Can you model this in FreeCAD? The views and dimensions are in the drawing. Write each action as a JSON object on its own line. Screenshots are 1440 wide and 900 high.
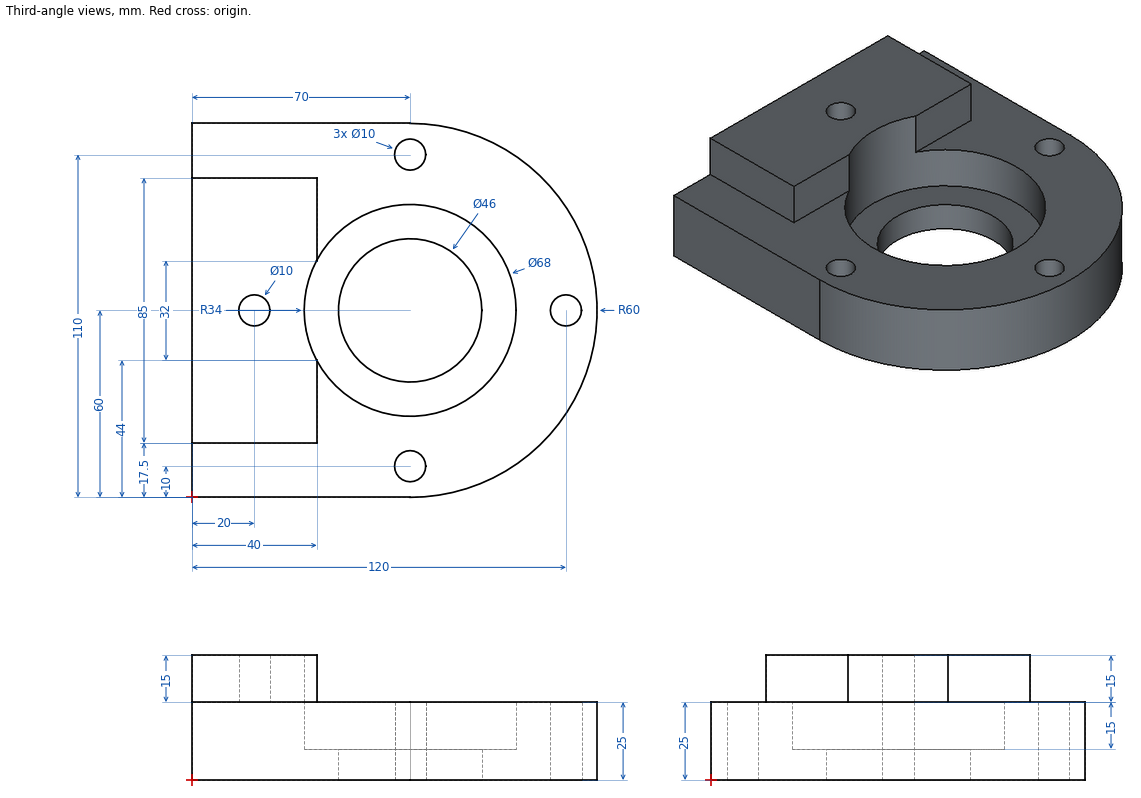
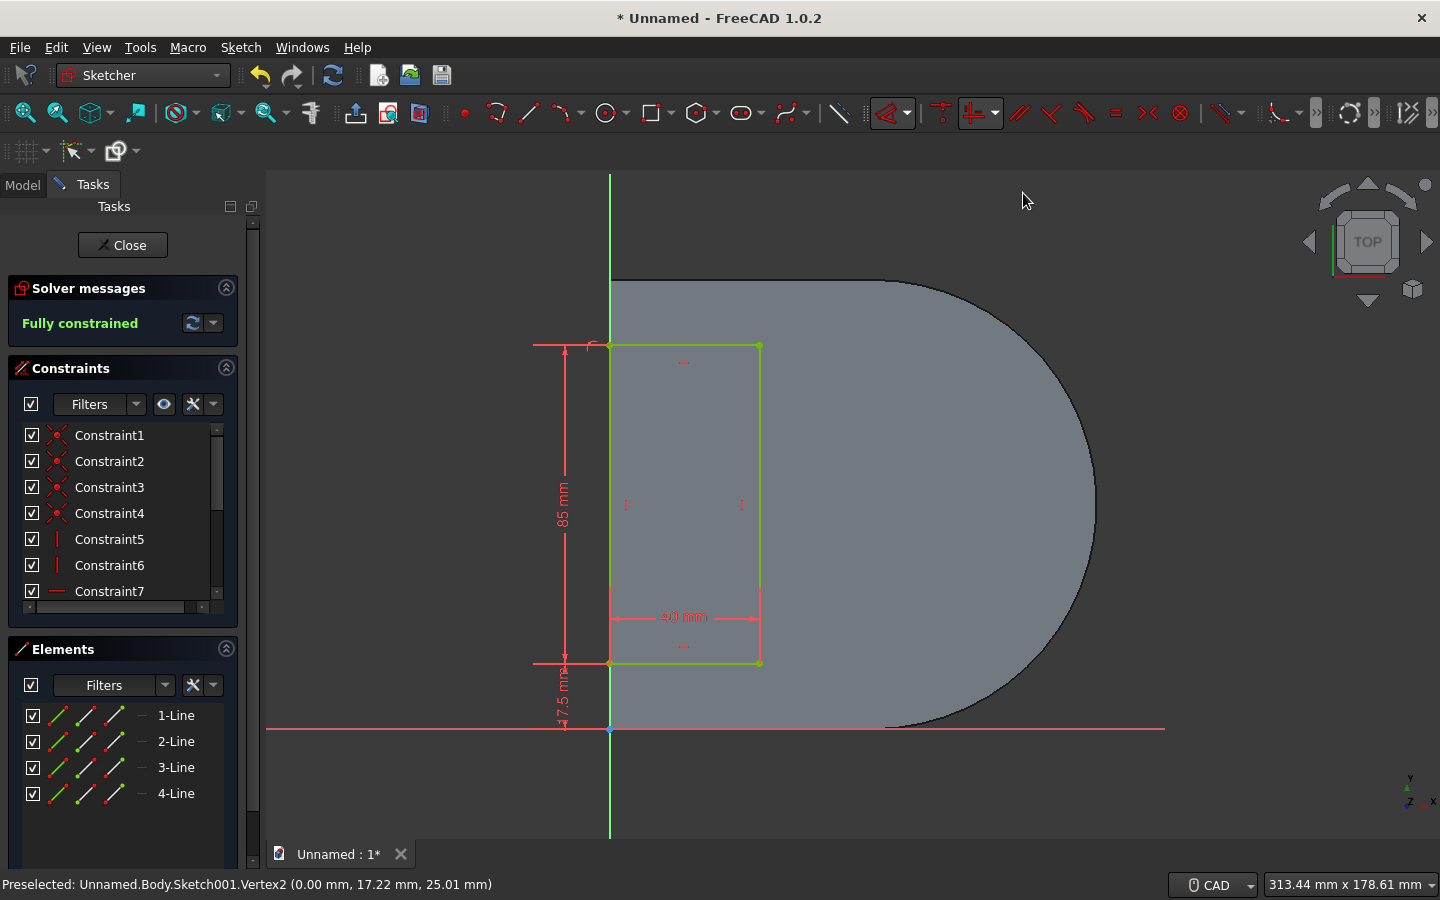
{"action": "left_click", "coordinate": [123, 245]}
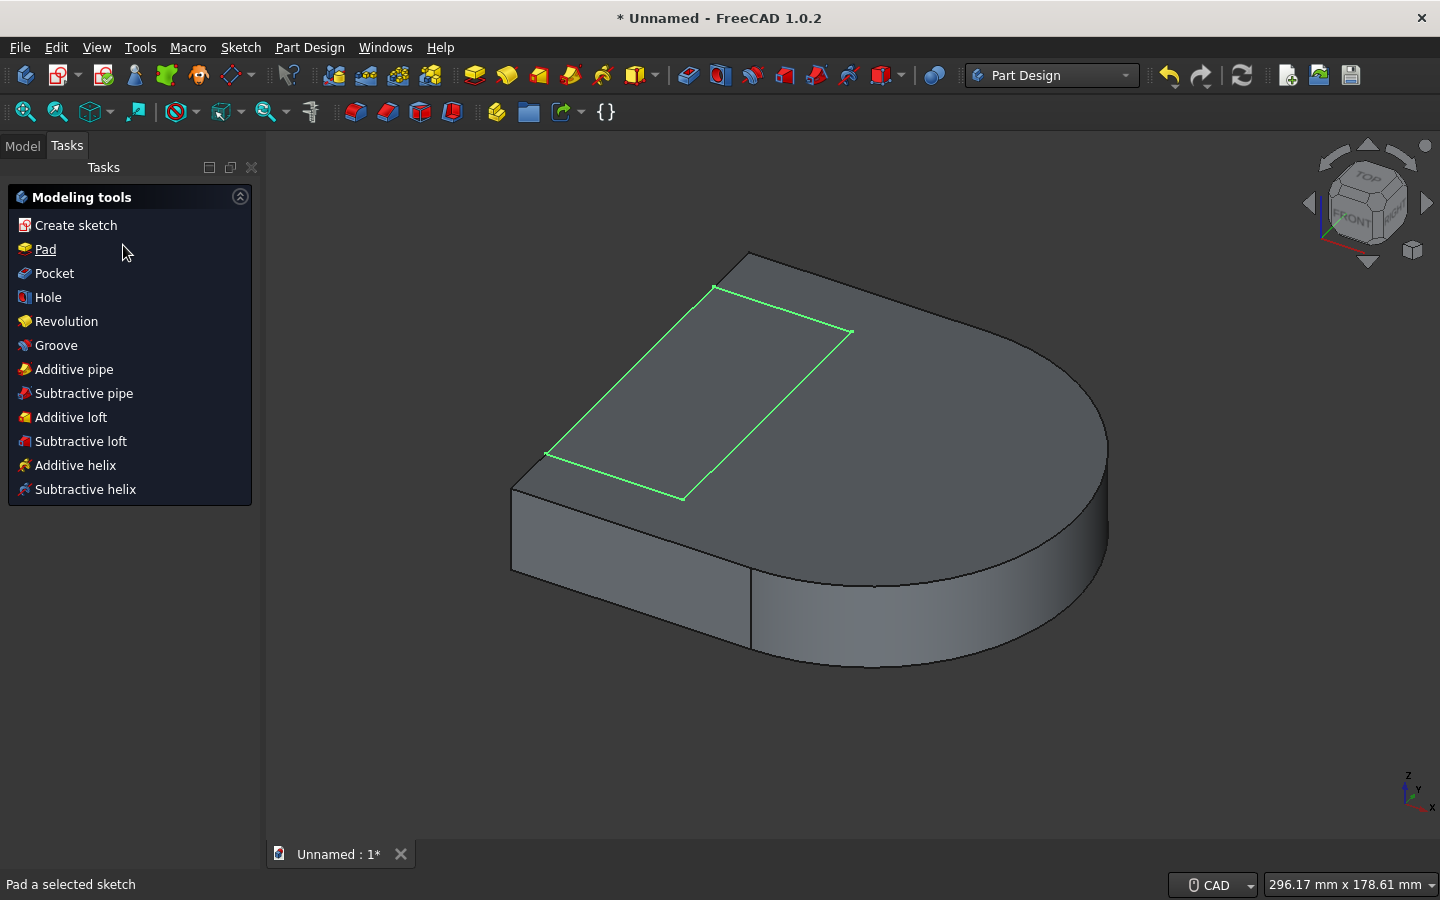
{"action": "left_click", "coordinate": [476, 76]}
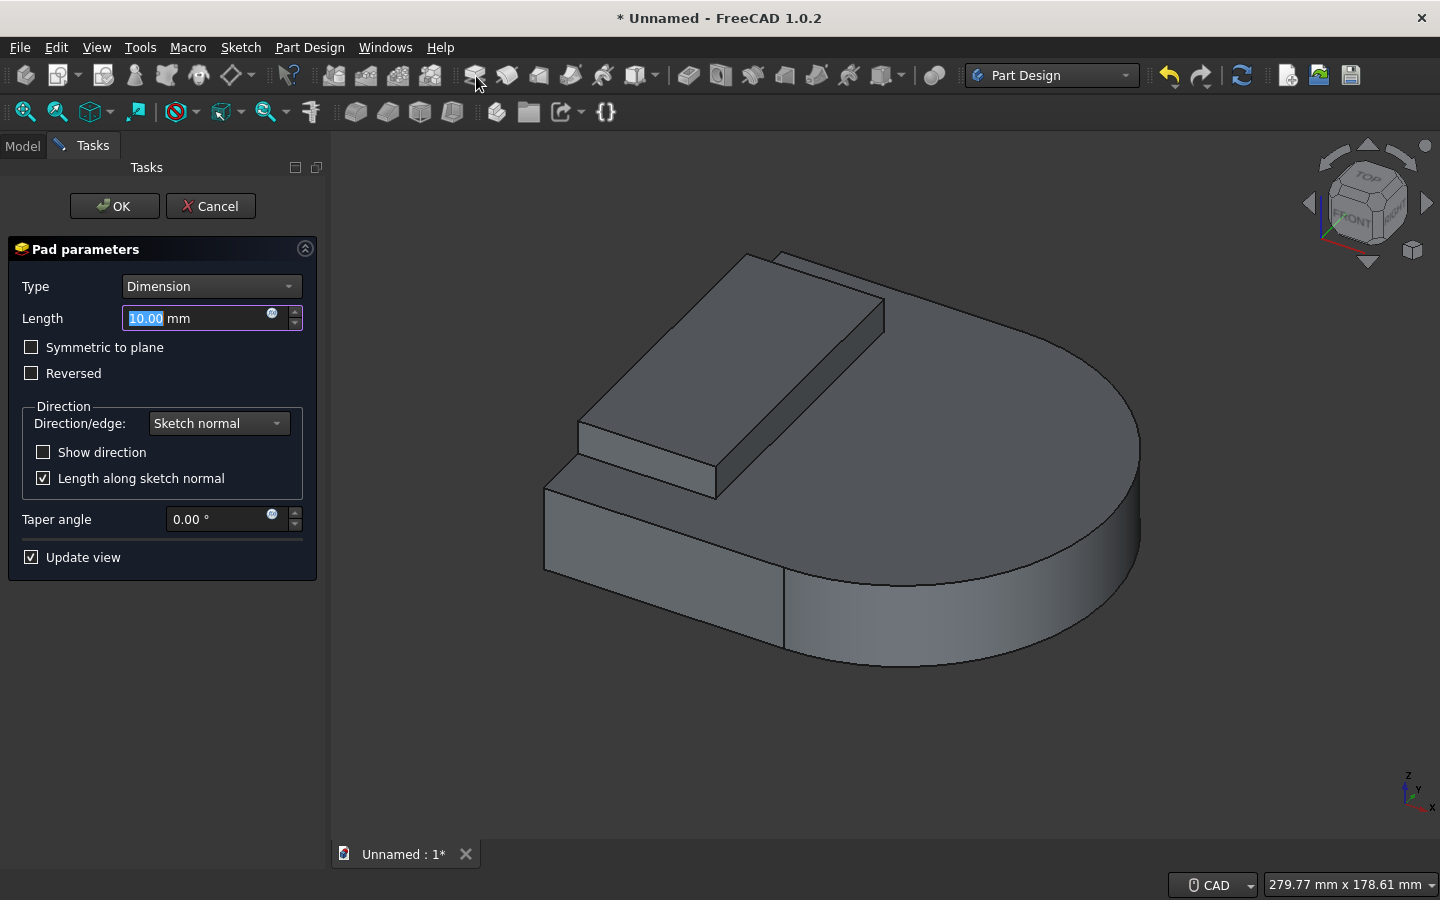
{"action": "type", "text": "15"}
{"action": "key", "text": "Tab"}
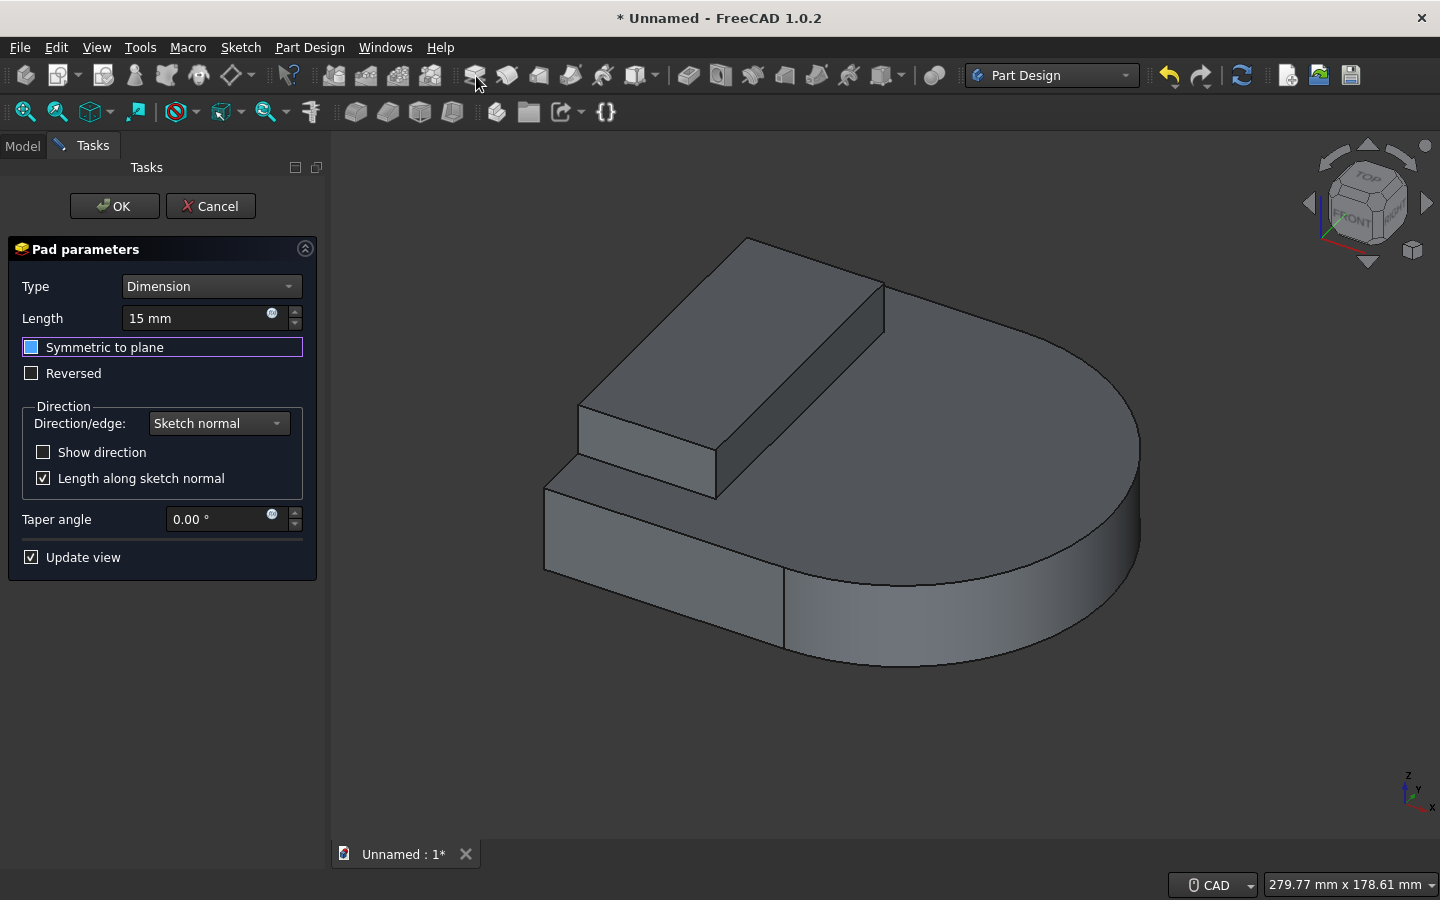
{"action": "left_click", "coordinate": [115, 206]}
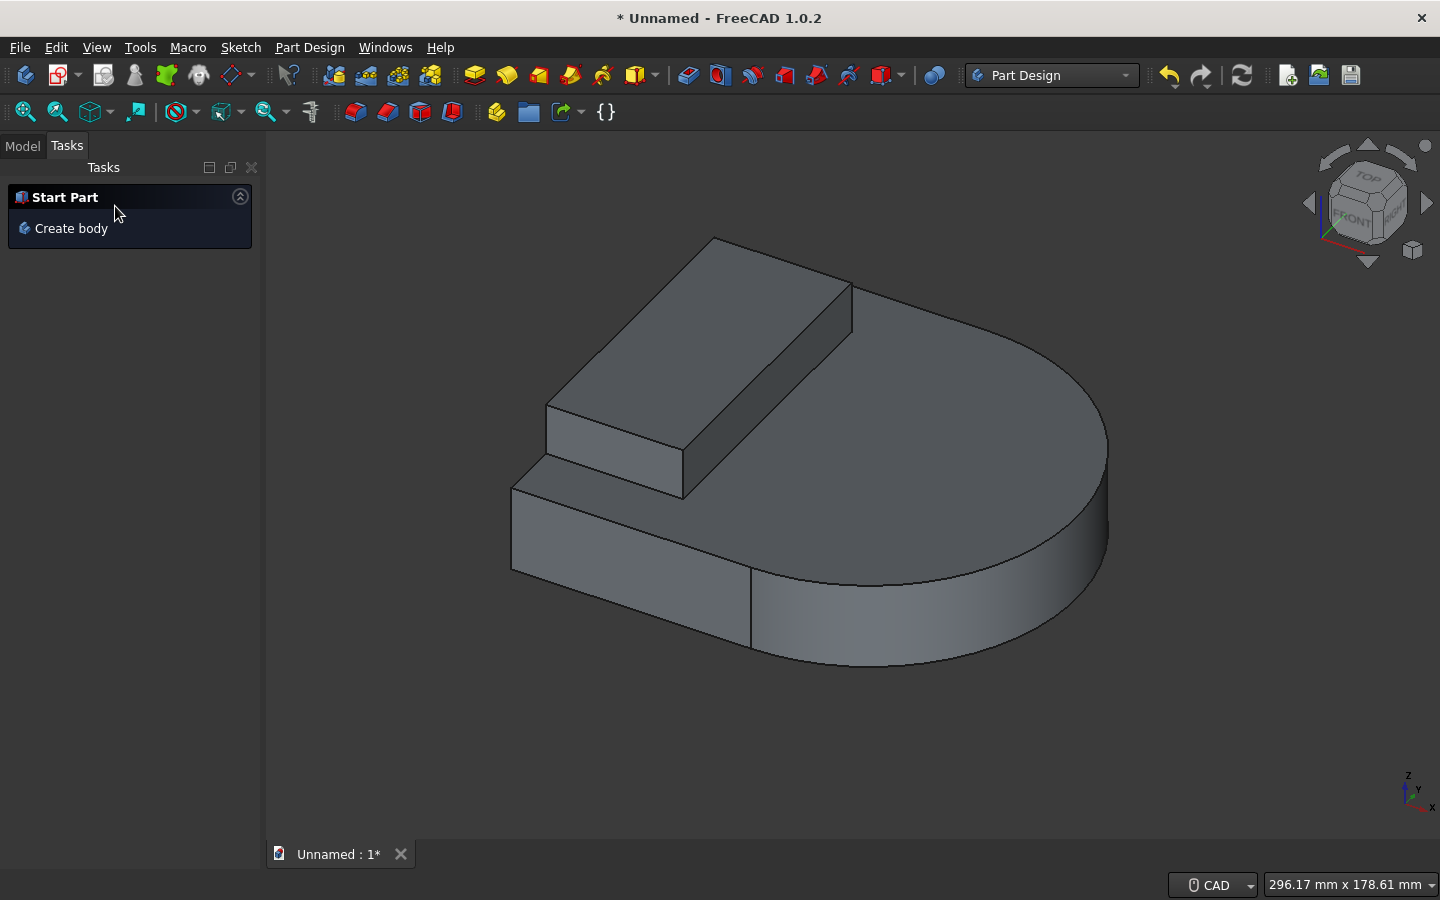
{"action": "left_click", "coordinate": [917, 464]}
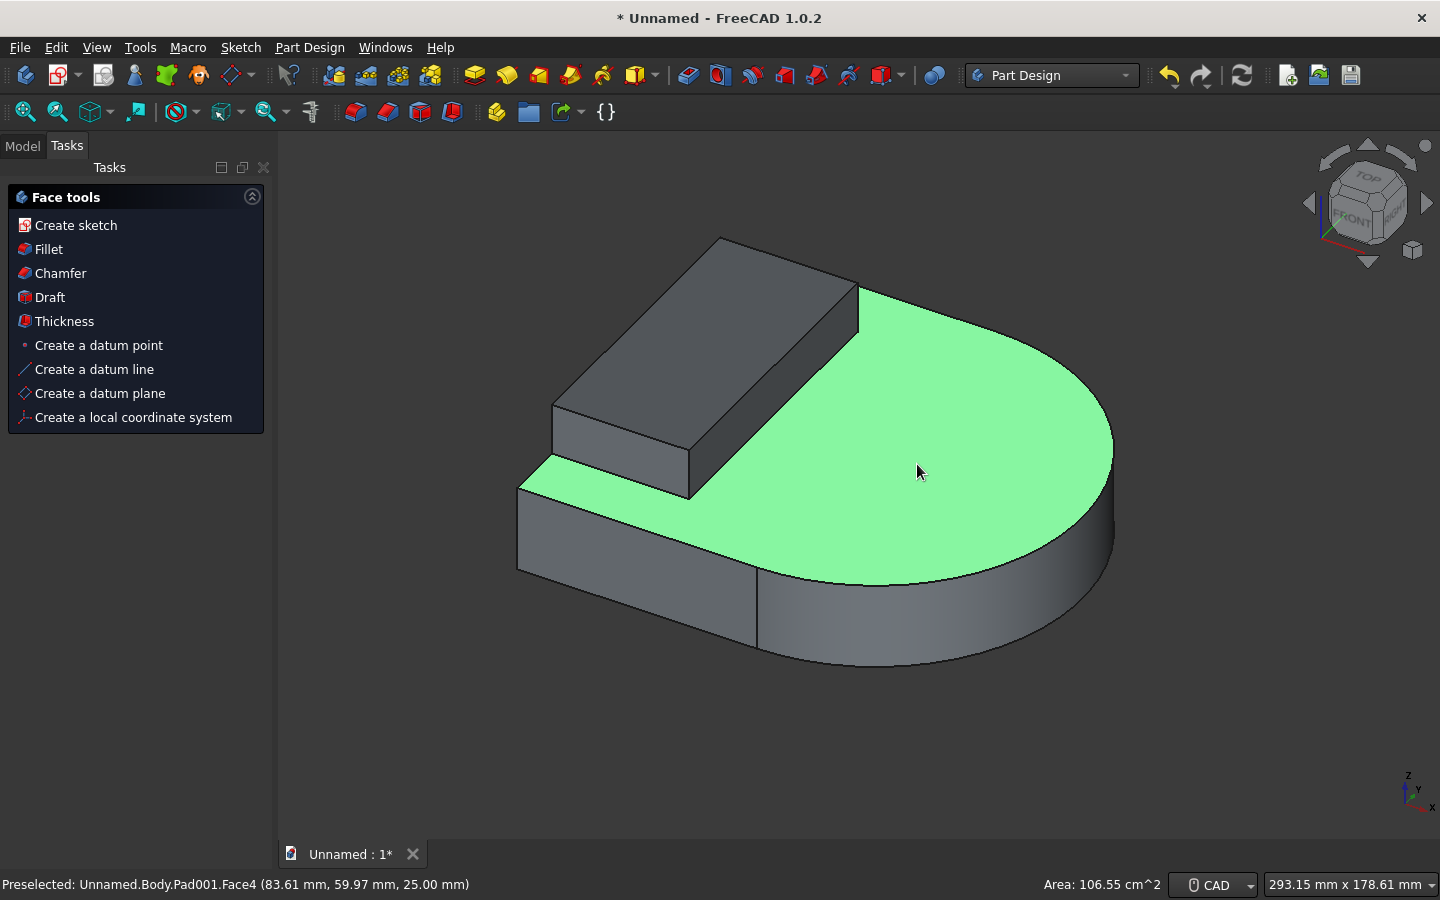
{"action": "left_click", "coordinate": [58, 76]}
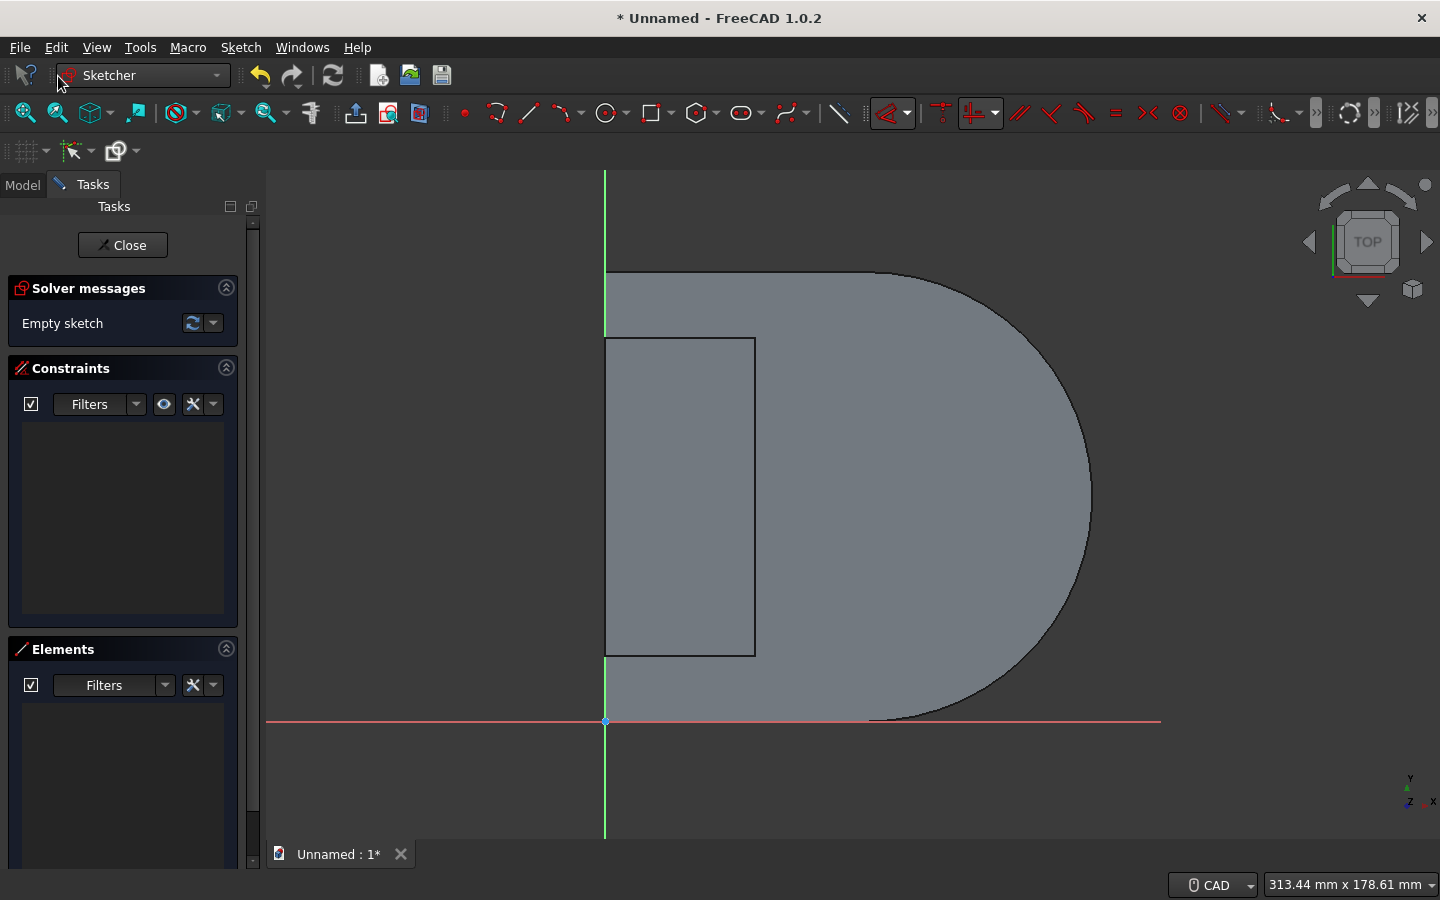
{"action": "left_click", "coordinate": [420, 114]}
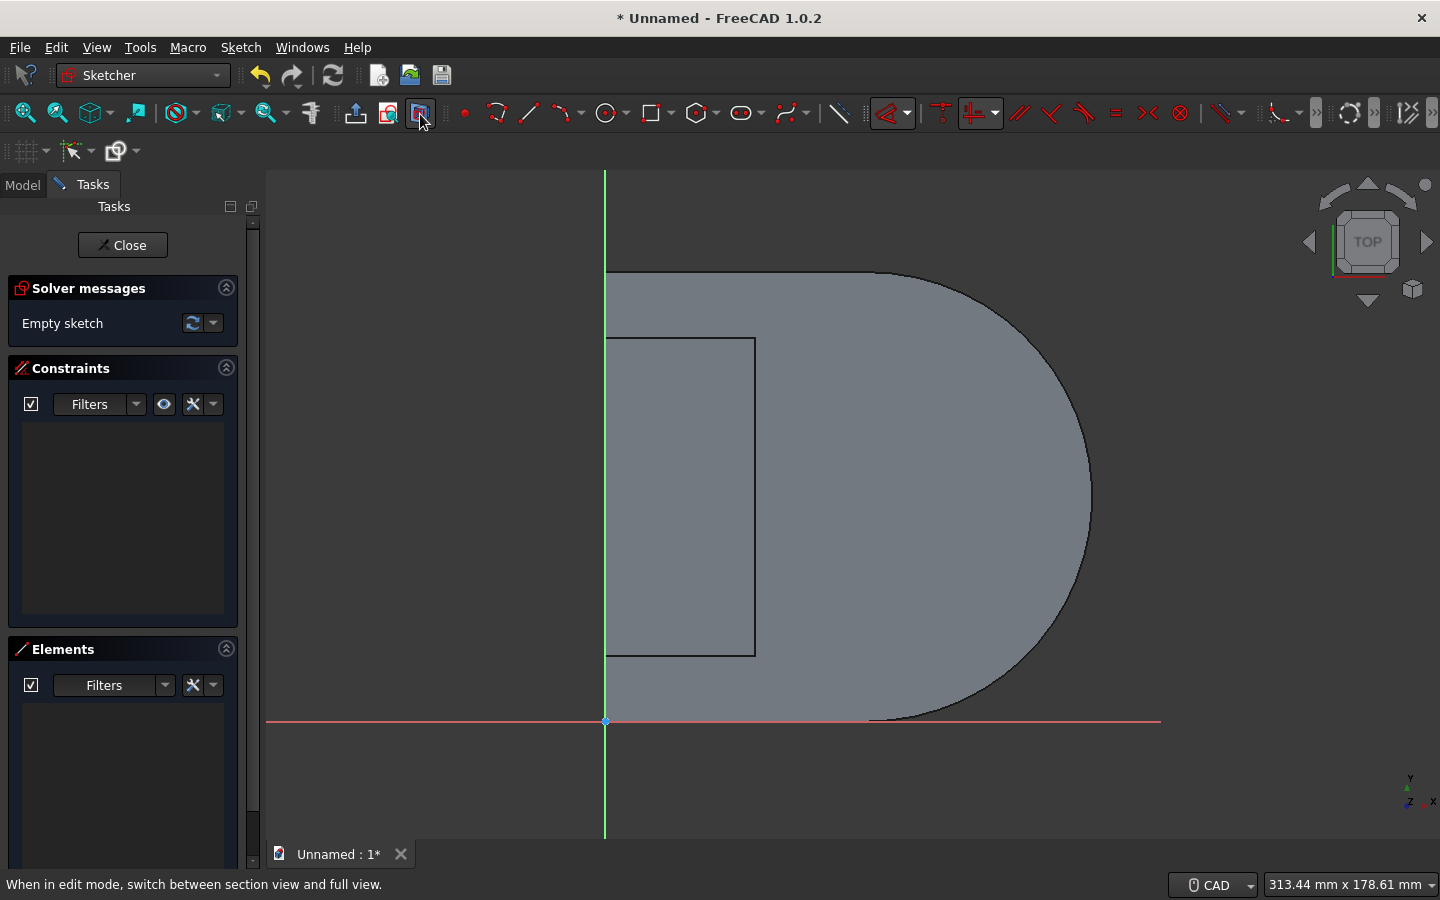
{"action": "left_click", "coordinate": [606, 114]}